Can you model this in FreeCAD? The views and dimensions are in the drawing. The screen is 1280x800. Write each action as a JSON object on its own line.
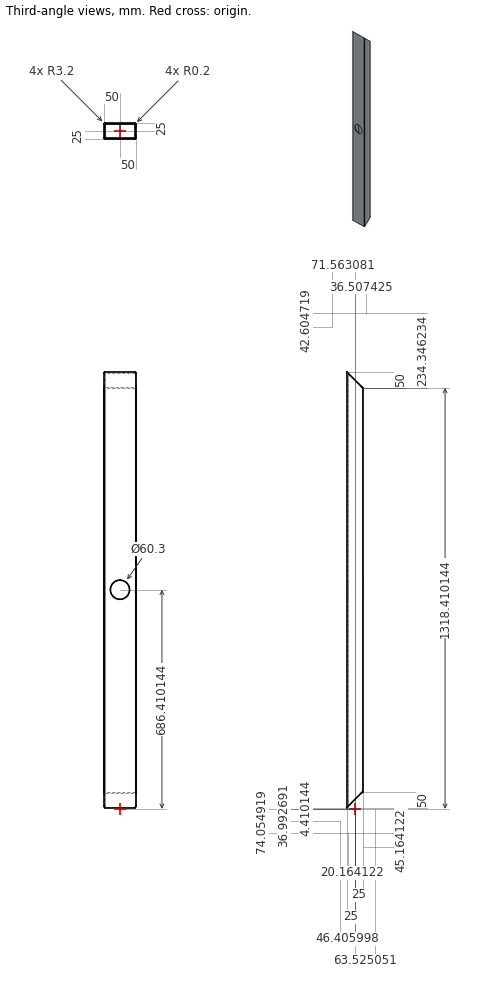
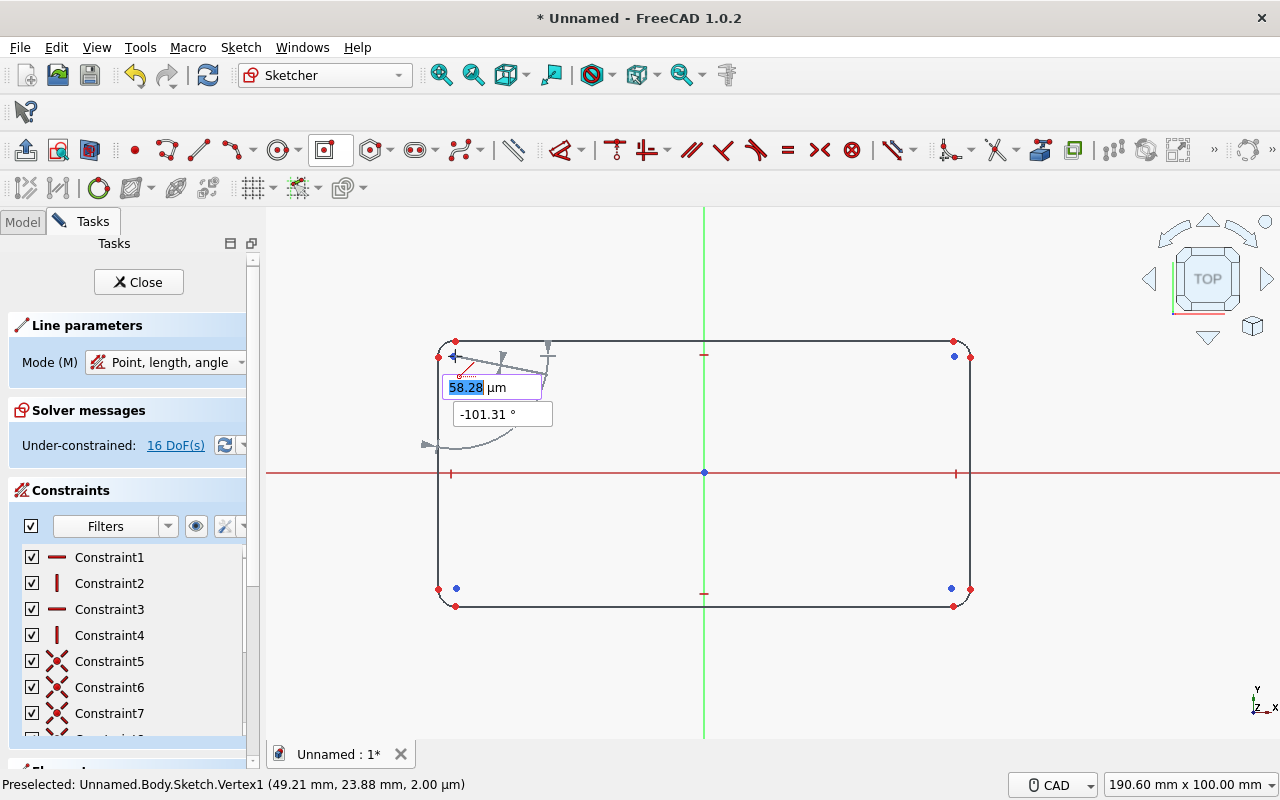
{"action": "scroll", "coordinate": [953, 356], "scroll_direction": "up", "scroll_amount": 14}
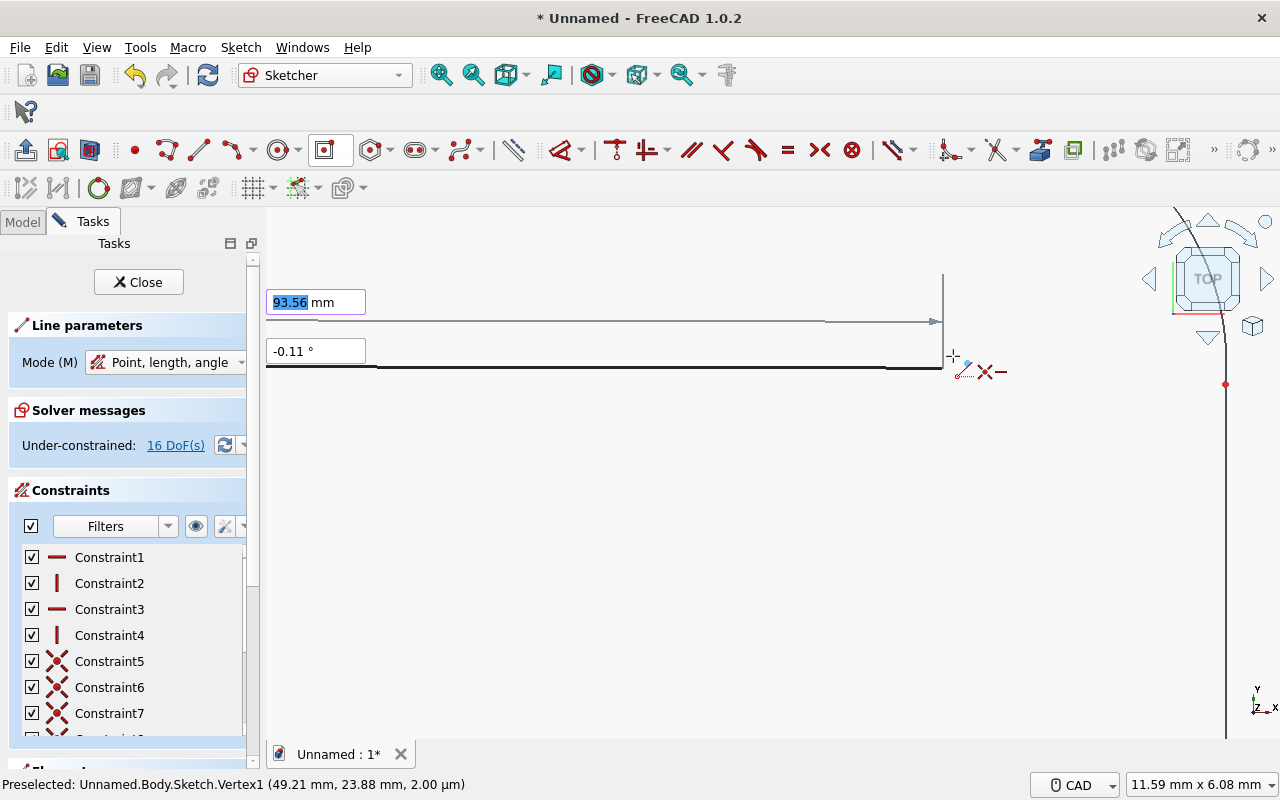
{"action": "left_click", "coordinate": [946, 351]}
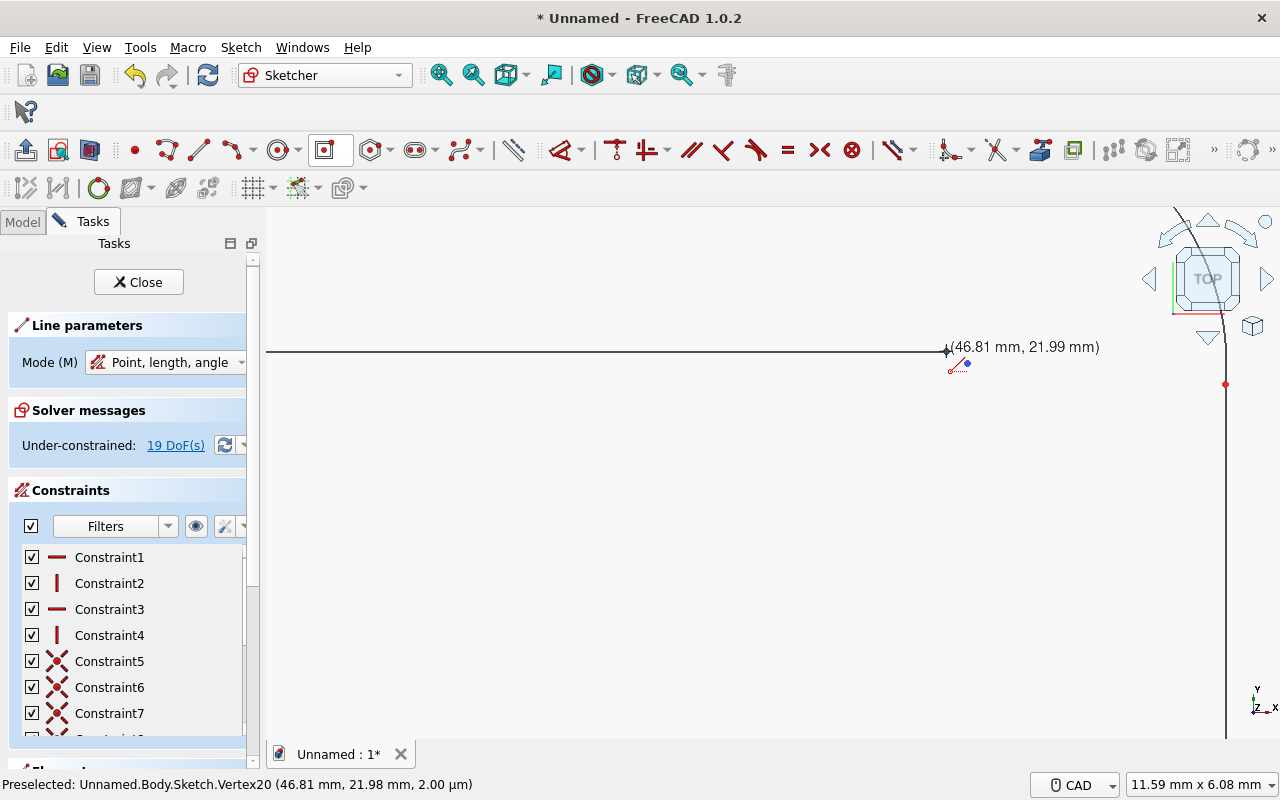
{"action": "left_click", "coordinate": [963, 369]}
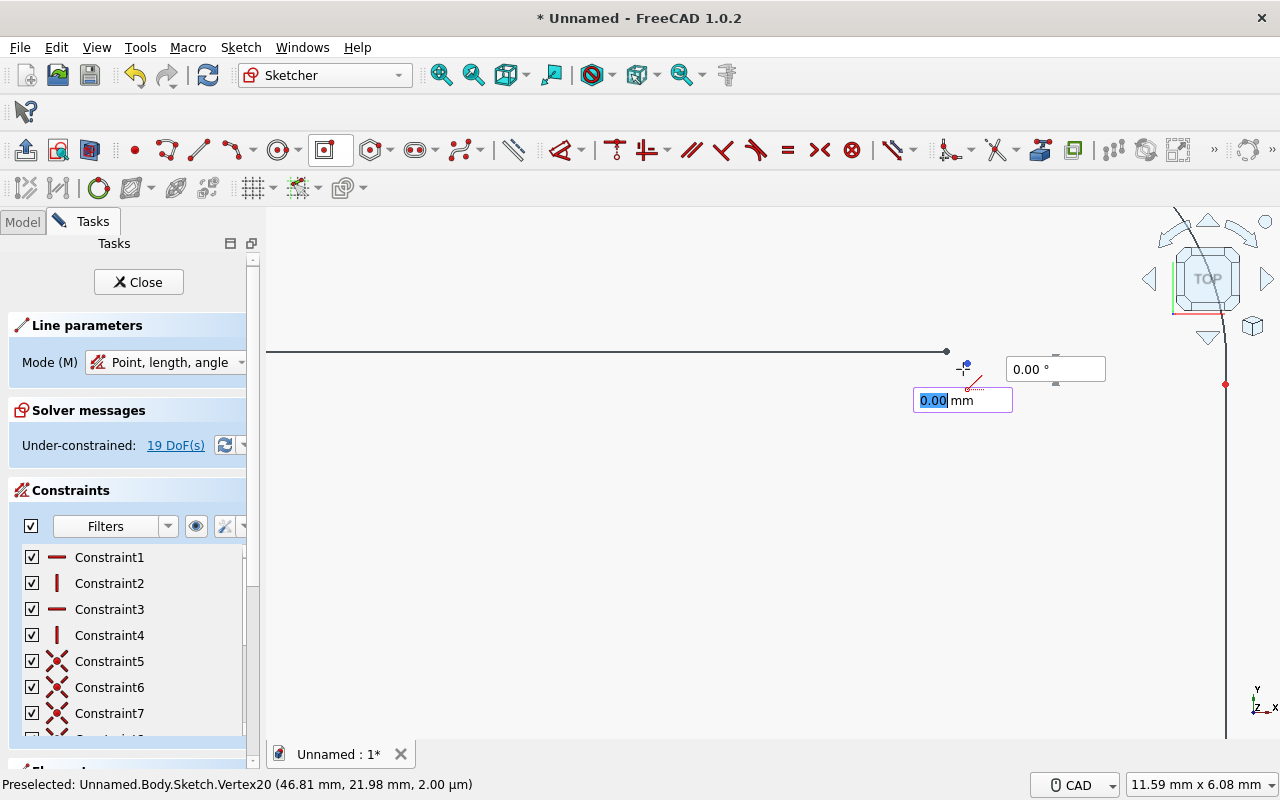
{"action": "scroll", "coordinate": [954, 356], "scroll_direction": "down", "scroll_amount": 14}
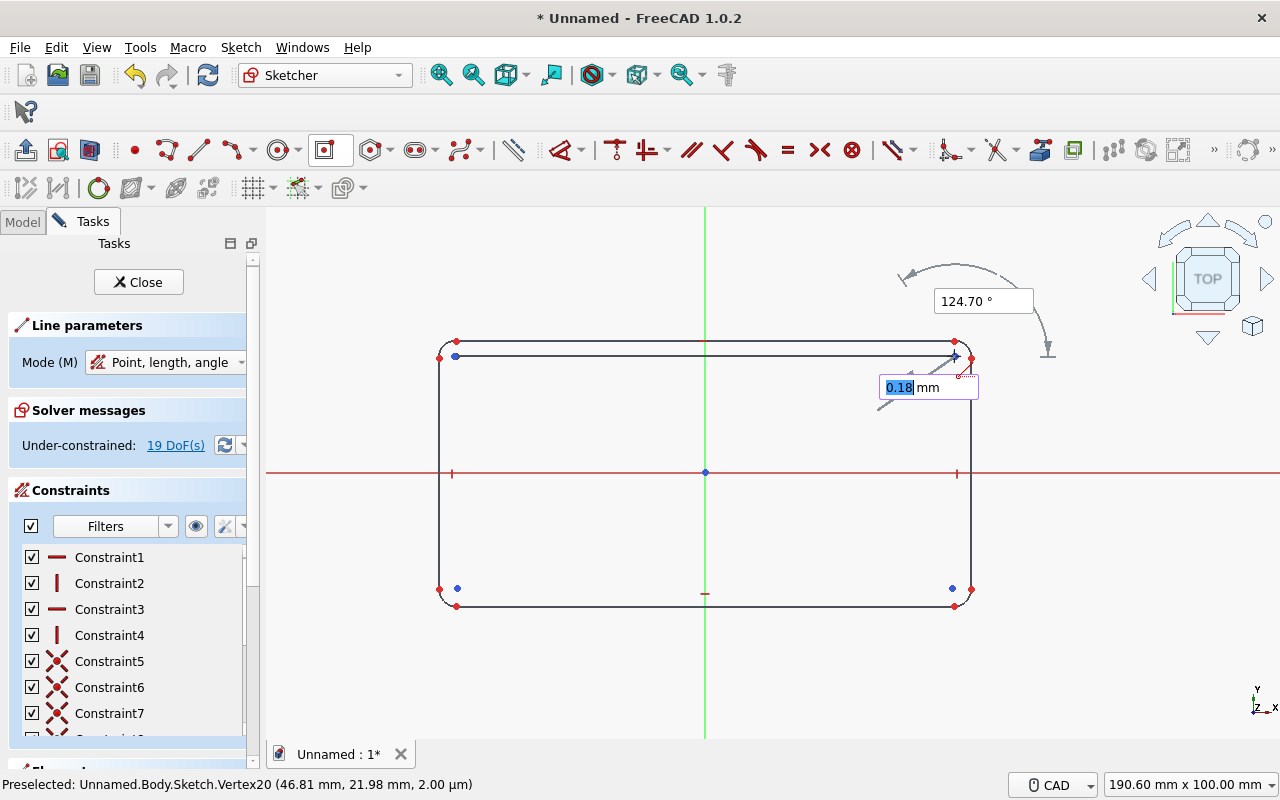
{"action": "scroll", "coordinate": [955, 589], "scroll_direction": "up", "scroll_amount": 14}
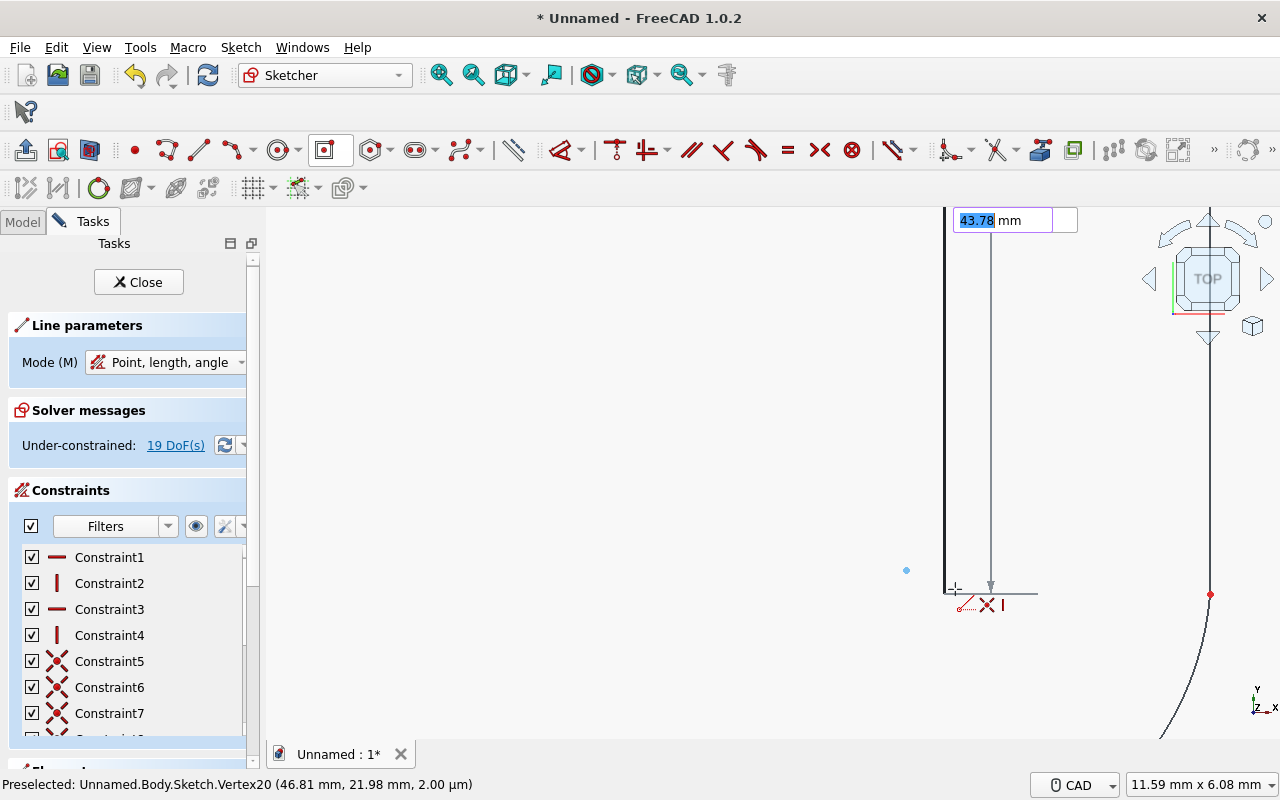
{"action": "left_click", "coordinate": [948, 577]}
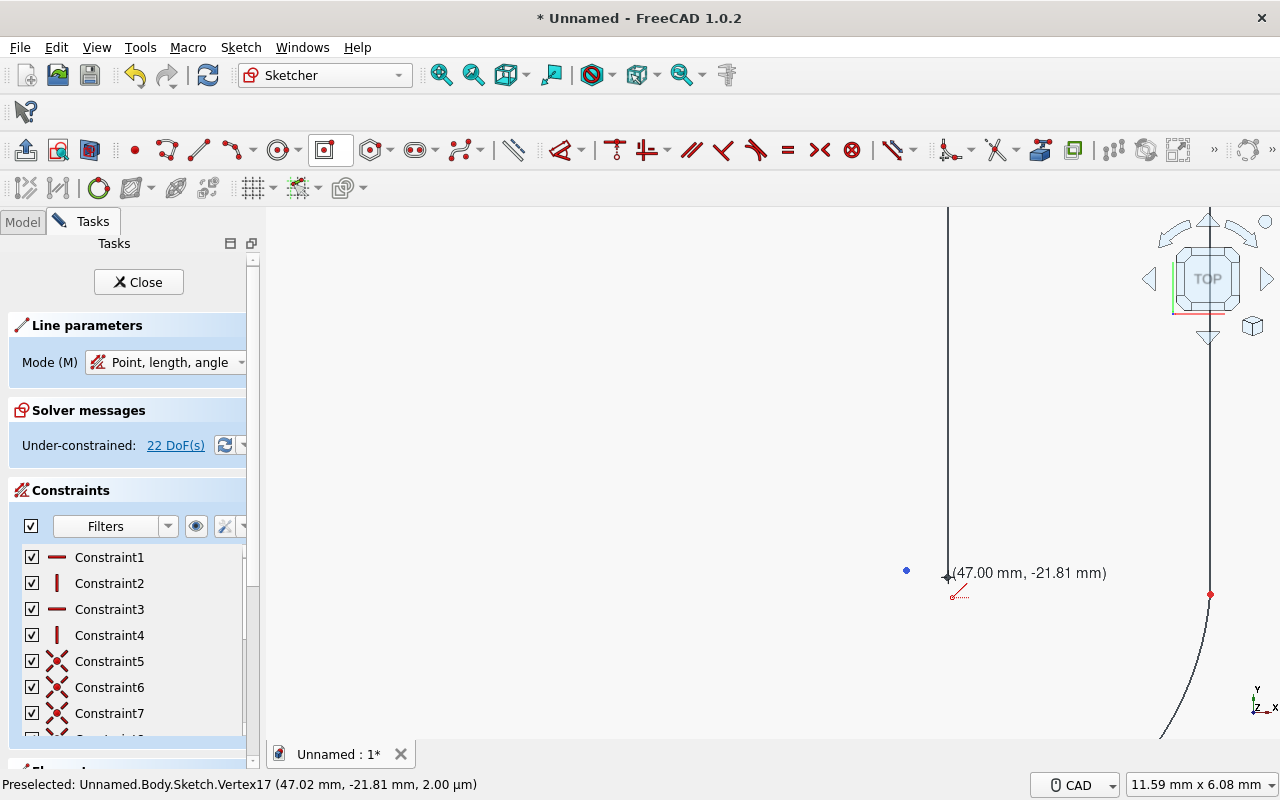
{"action": "left_click", "coordinate": [930, 595]}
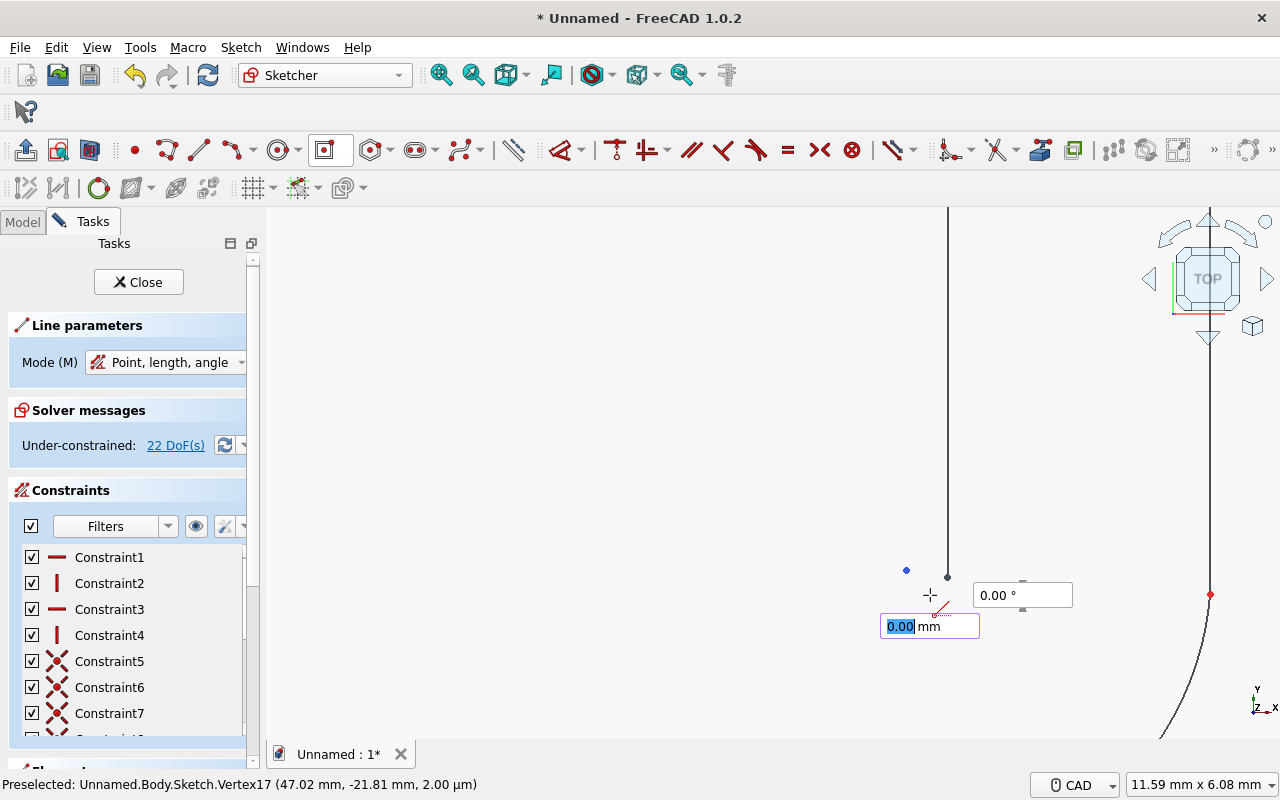
{"action": "scroll", "coordinate": [955, 590], "scroll_direction": "down", "scroll_amount": 14}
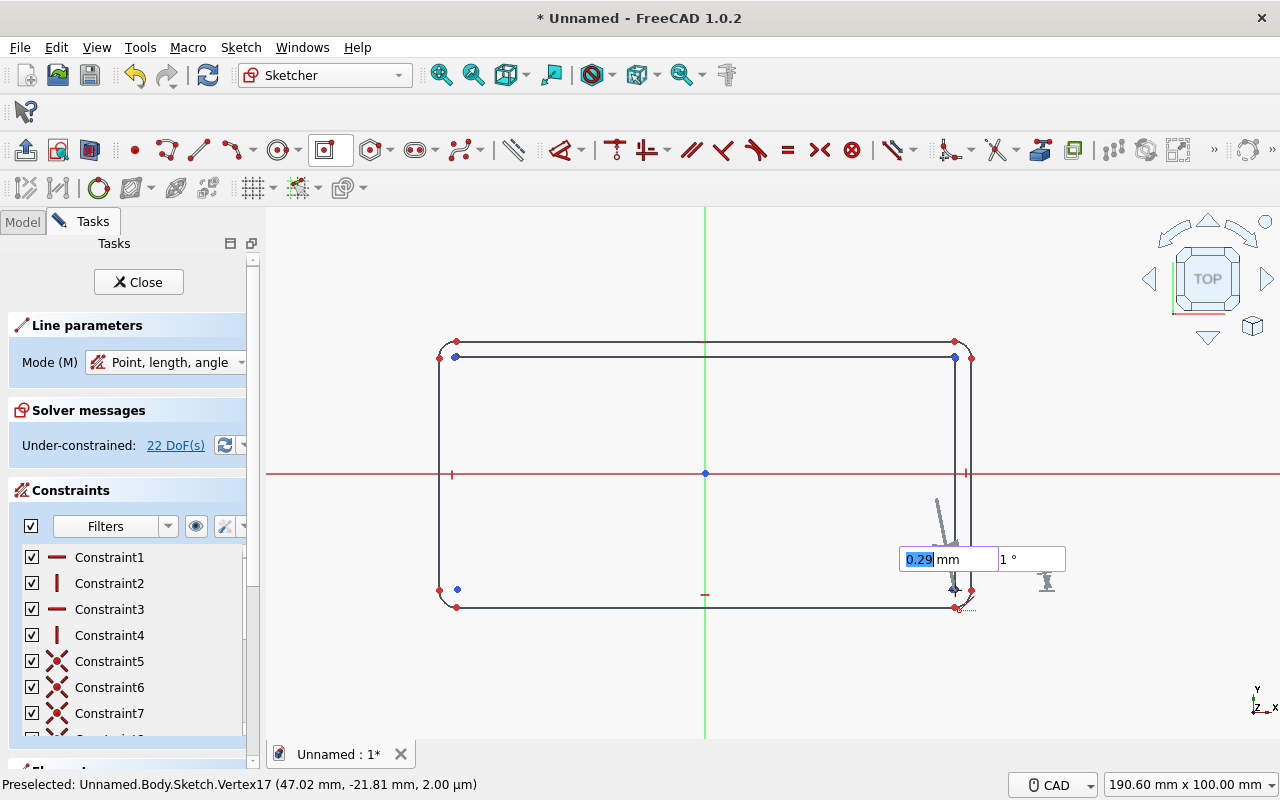
{"action": "scroll", "coordinate": [456, 591], "scroll_direction": "up", "scroll_amount": 14}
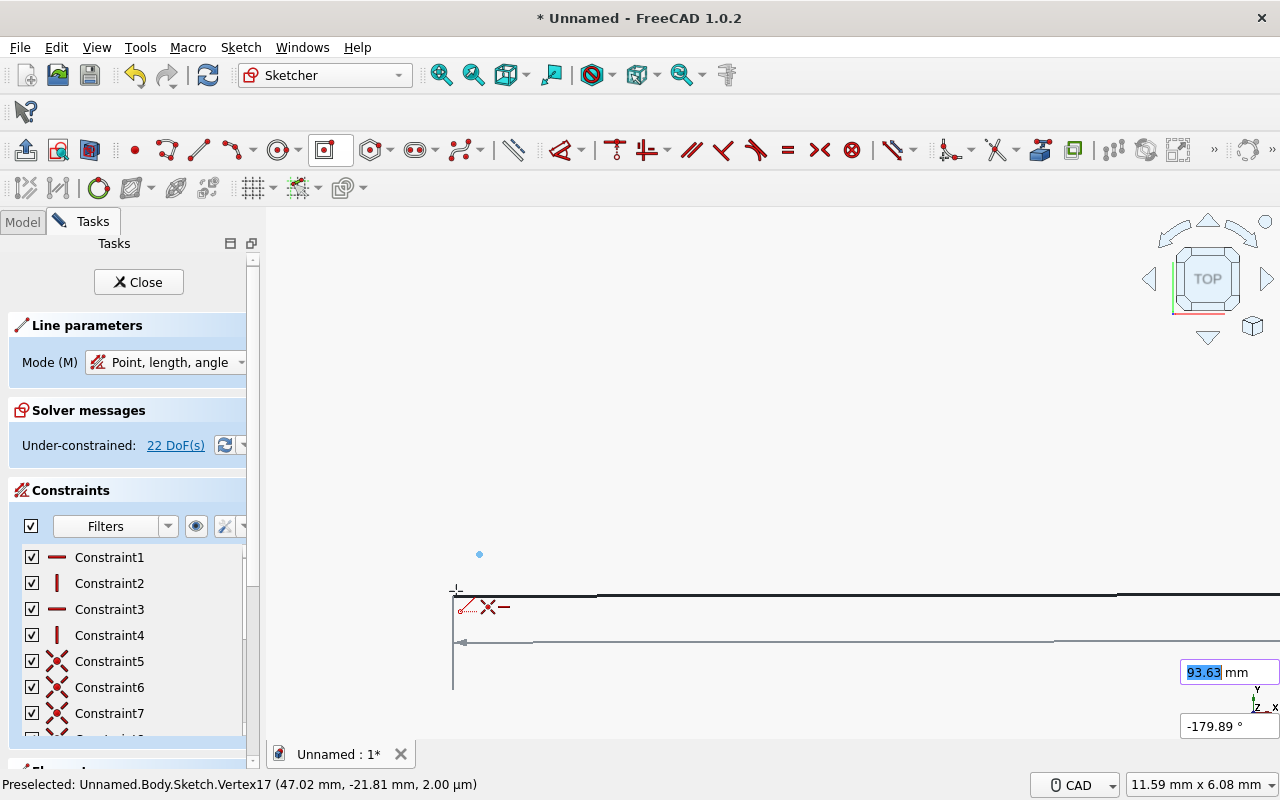
{"action": "left_click", "coordinate": [456, 580]}